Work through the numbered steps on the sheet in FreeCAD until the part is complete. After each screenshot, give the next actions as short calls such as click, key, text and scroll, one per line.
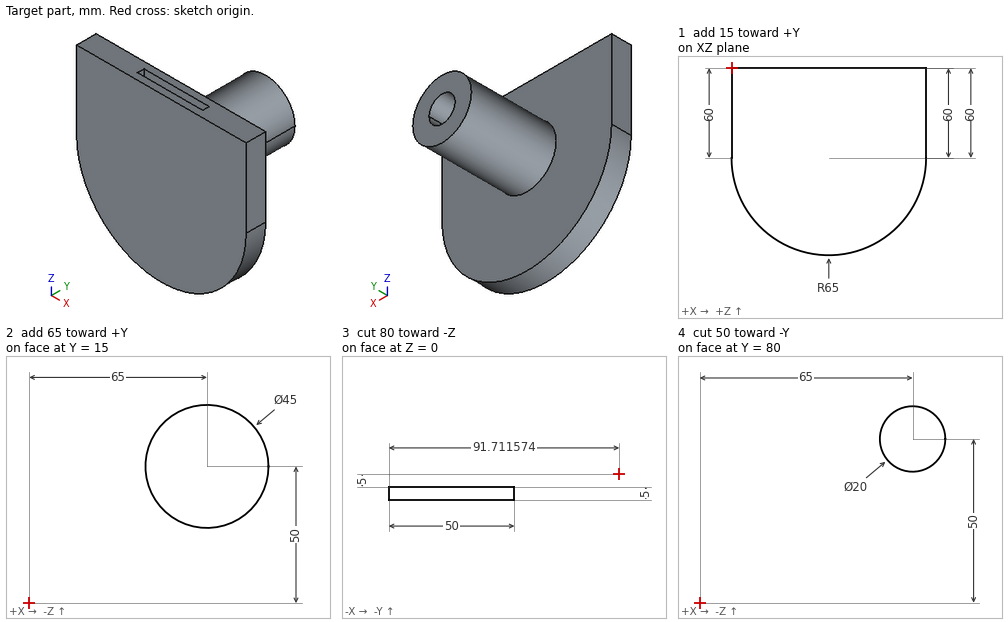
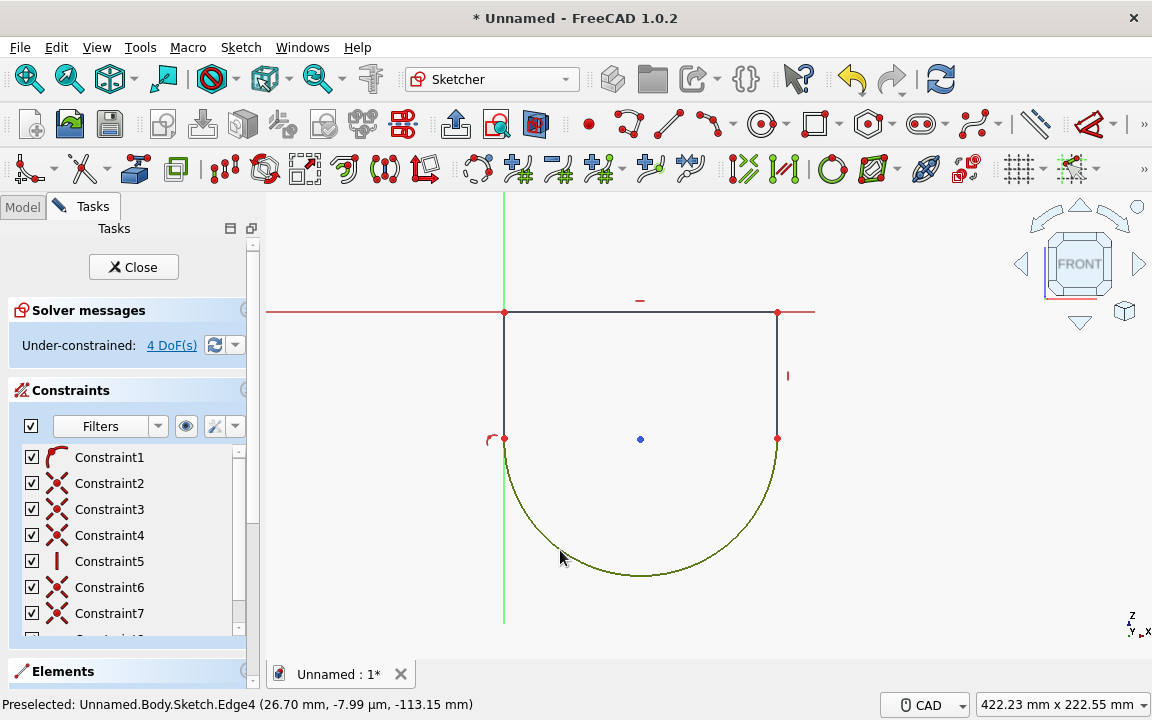
key(k)
key(r)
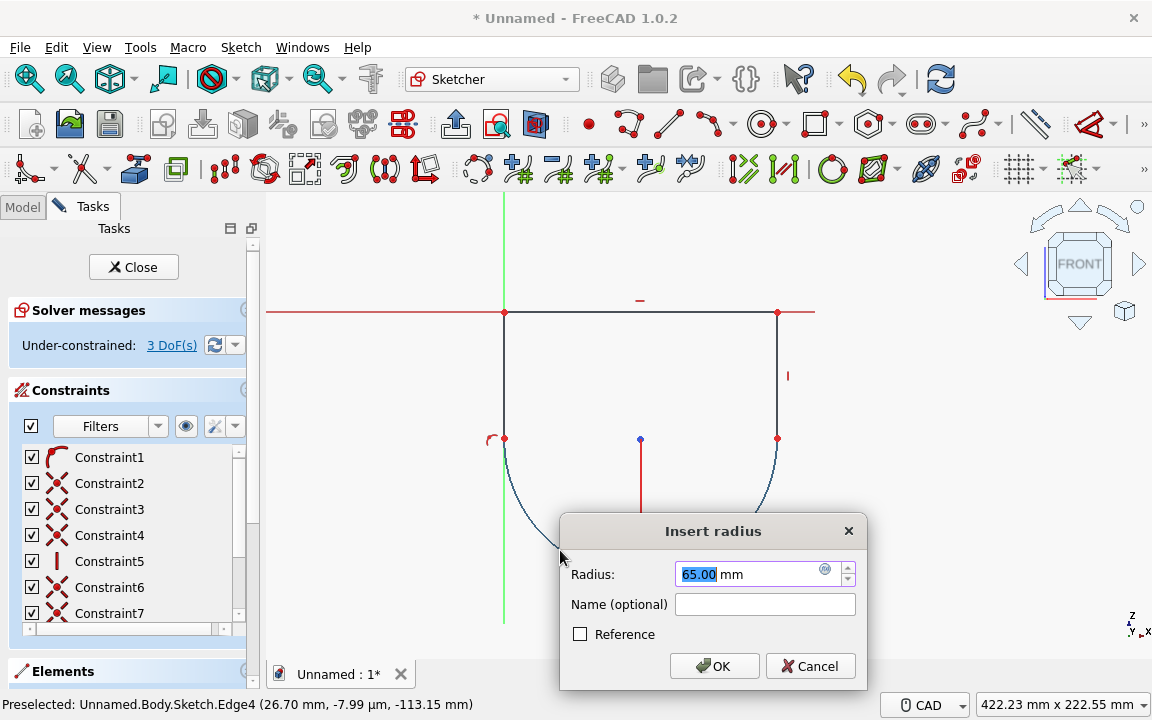
text(65)
key(Return)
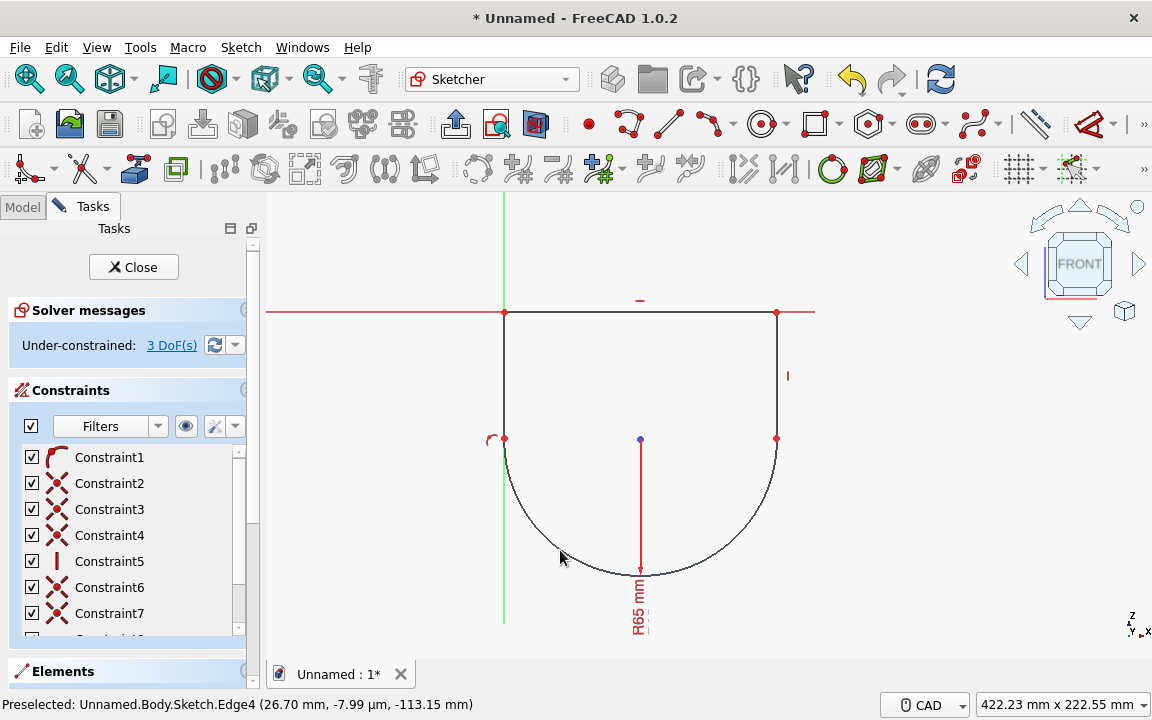
click(504, 401)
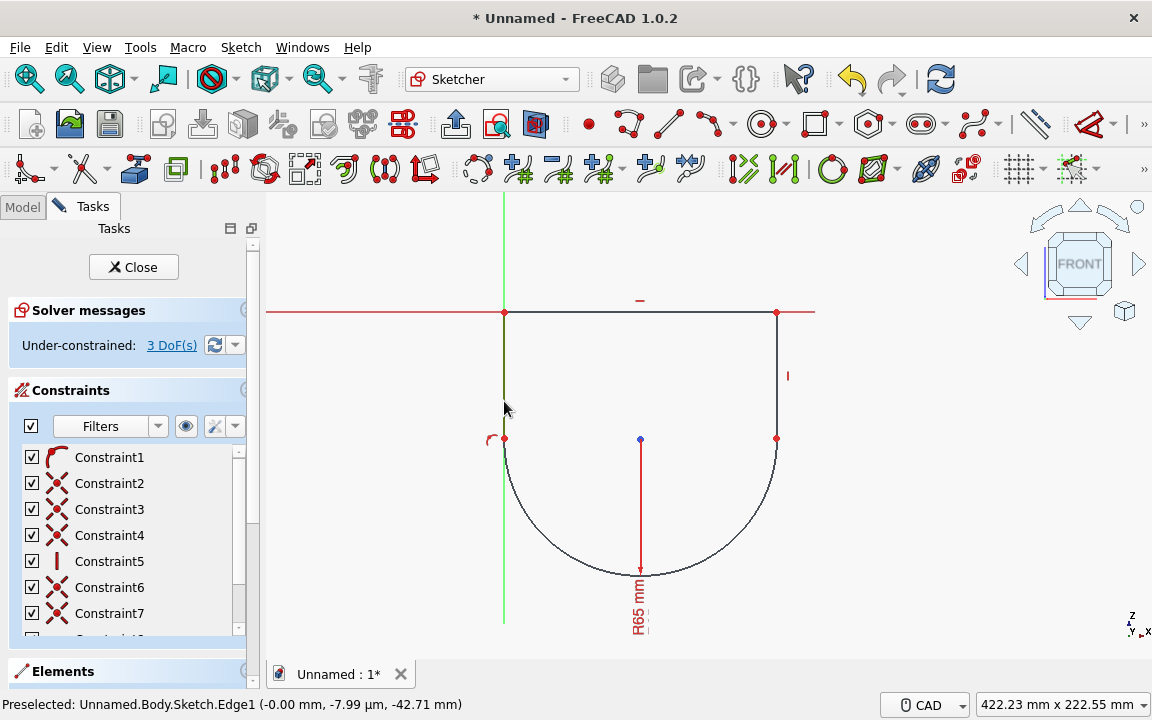
click(1116, 124)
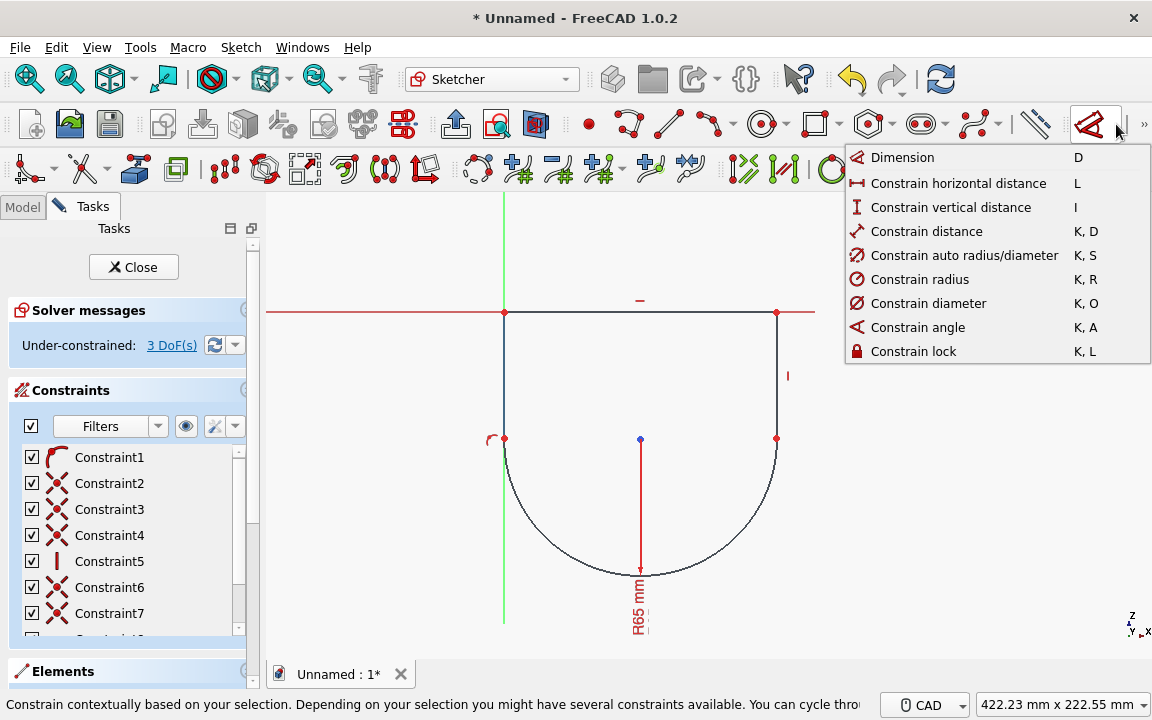
click(998, 207)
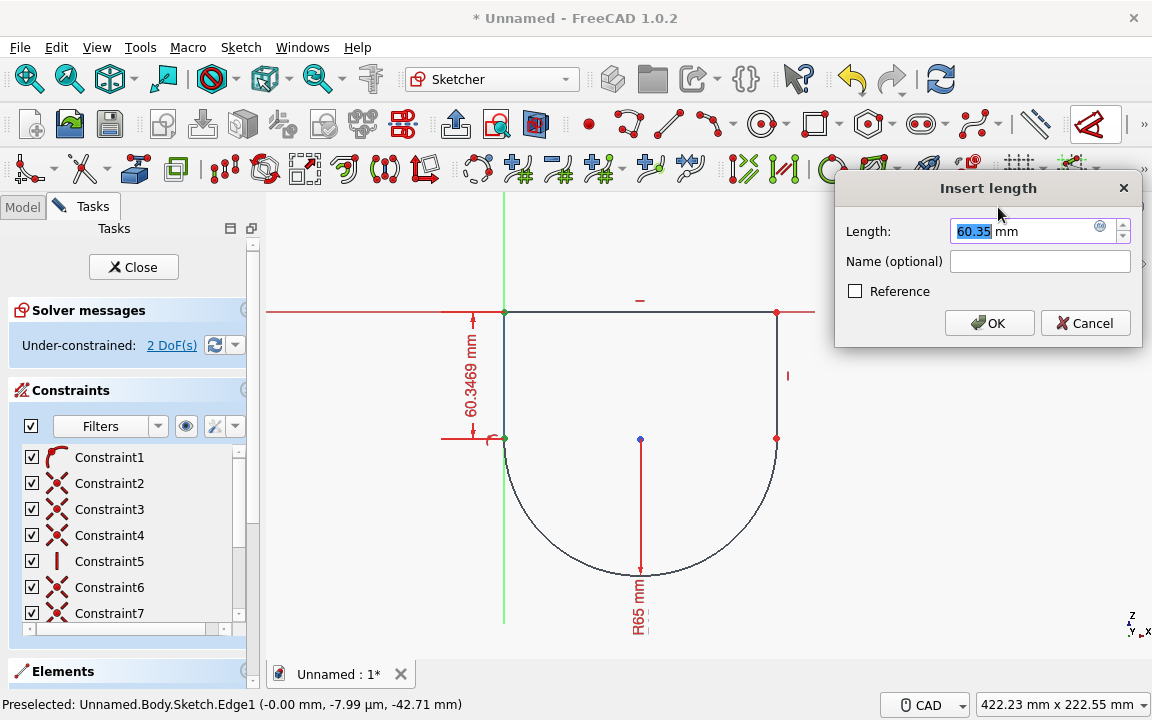
text(60)
key(Return)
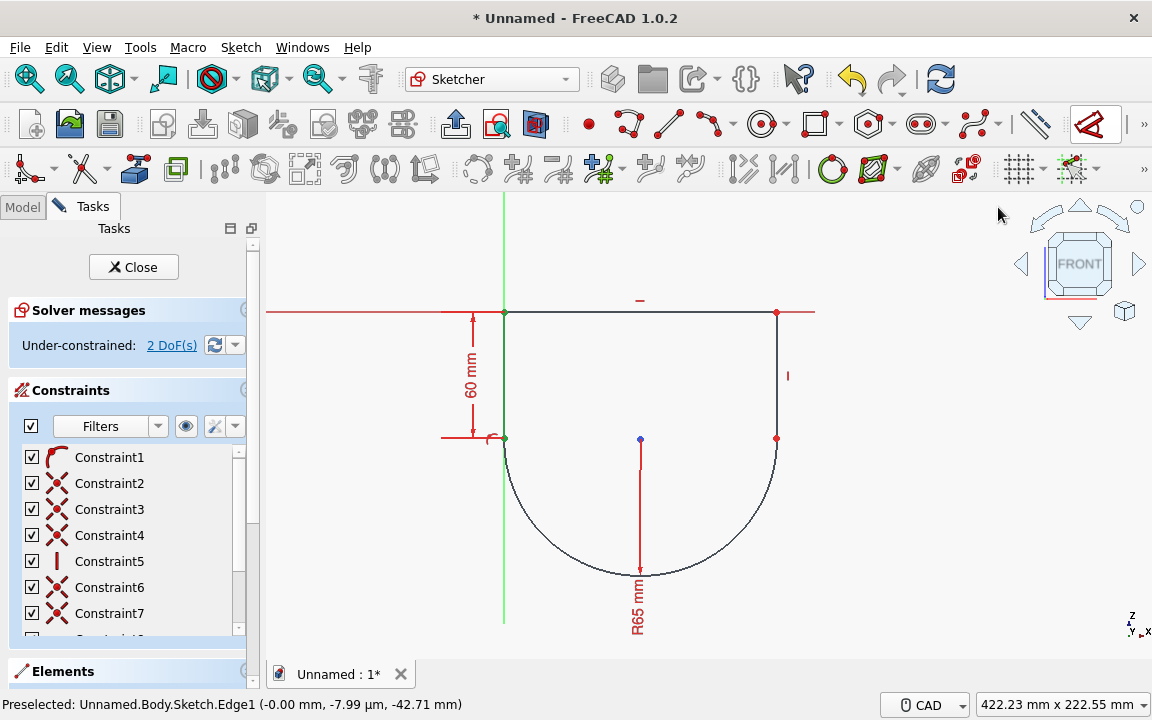
click(777, 350)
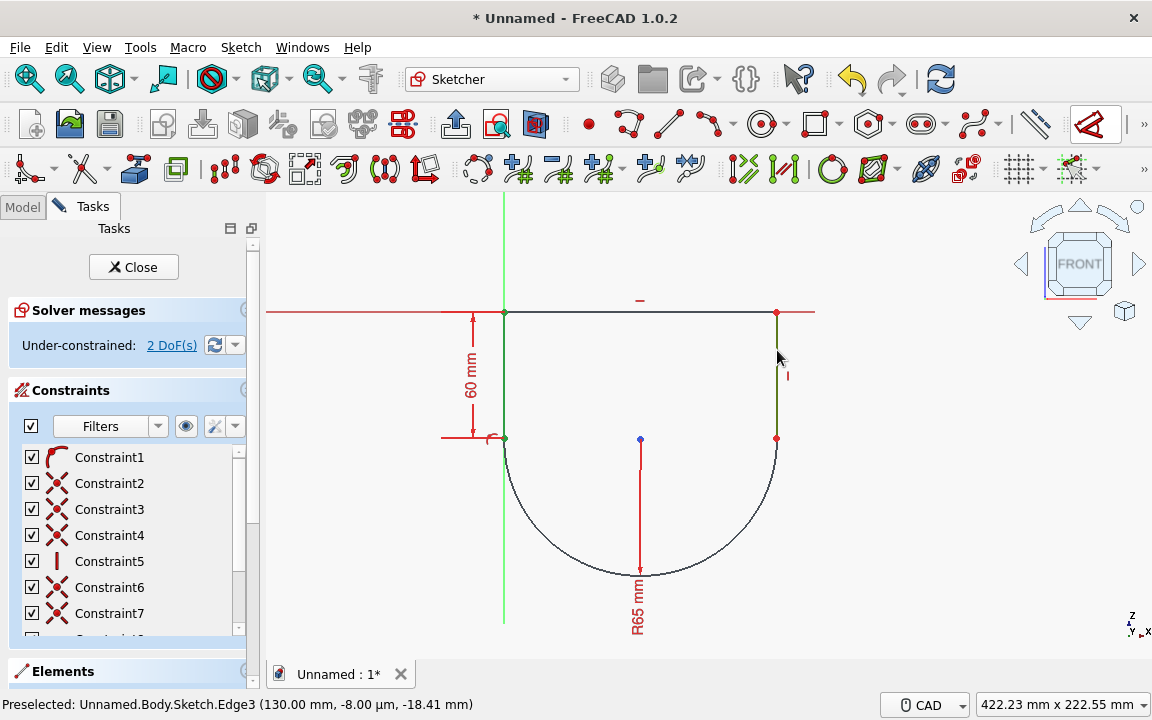
key(i)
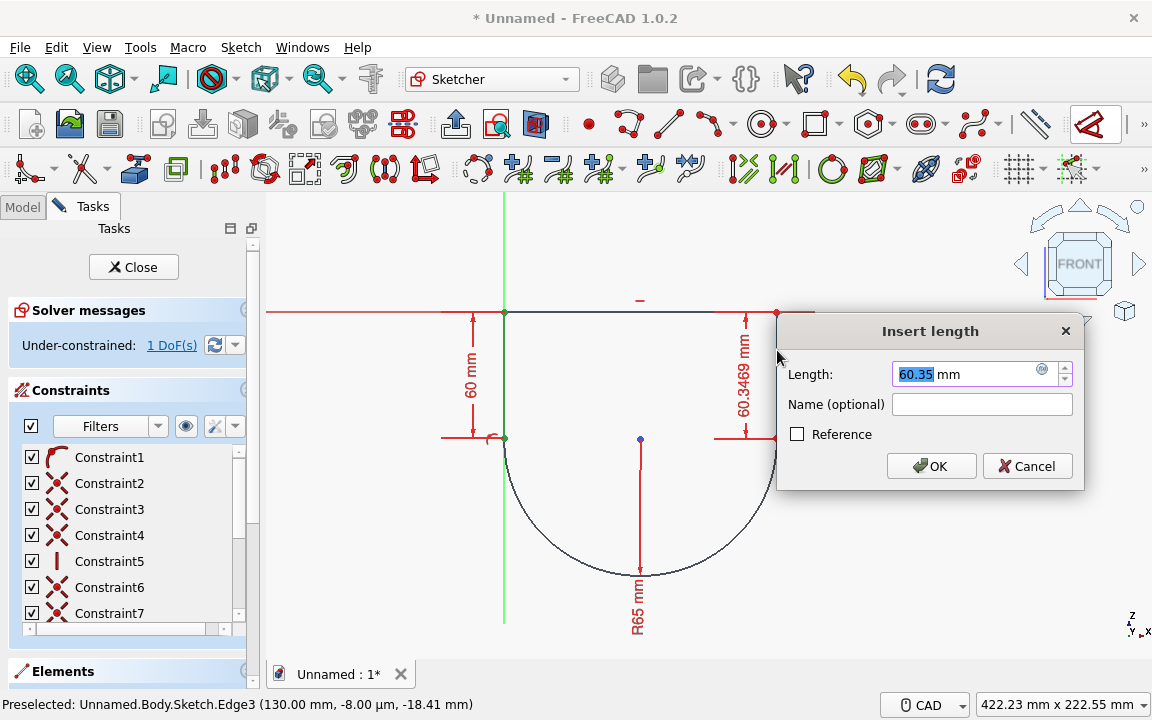
text(60)
key(Return)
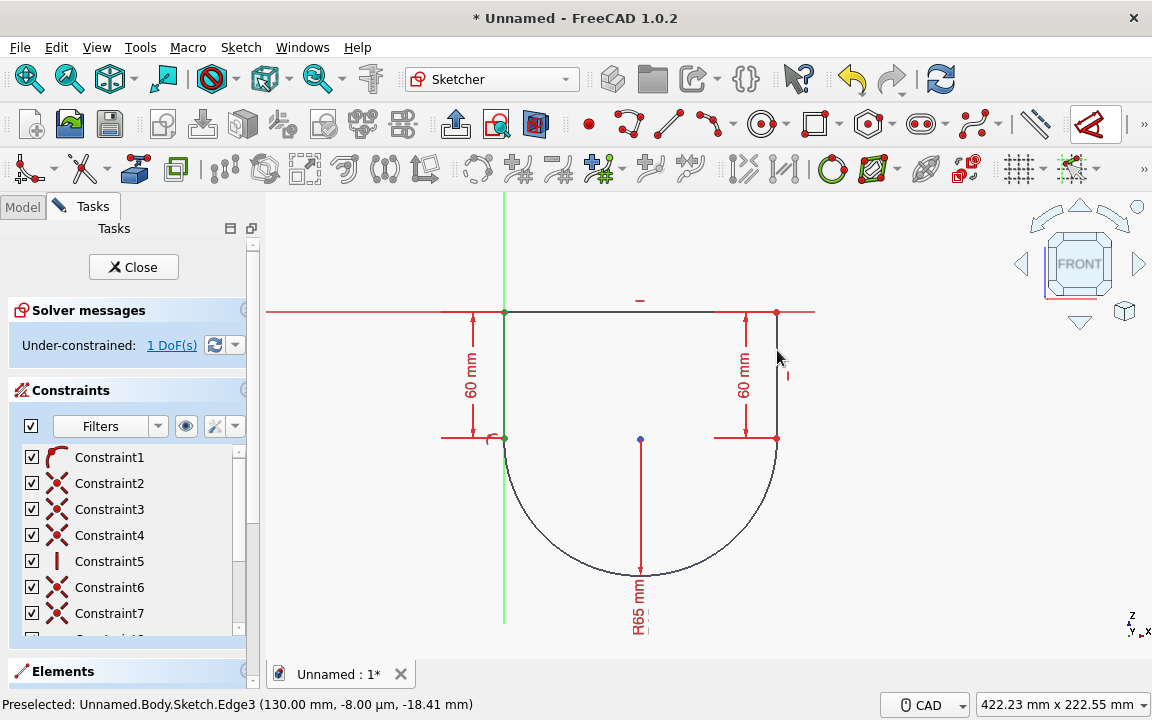
click(641, 440)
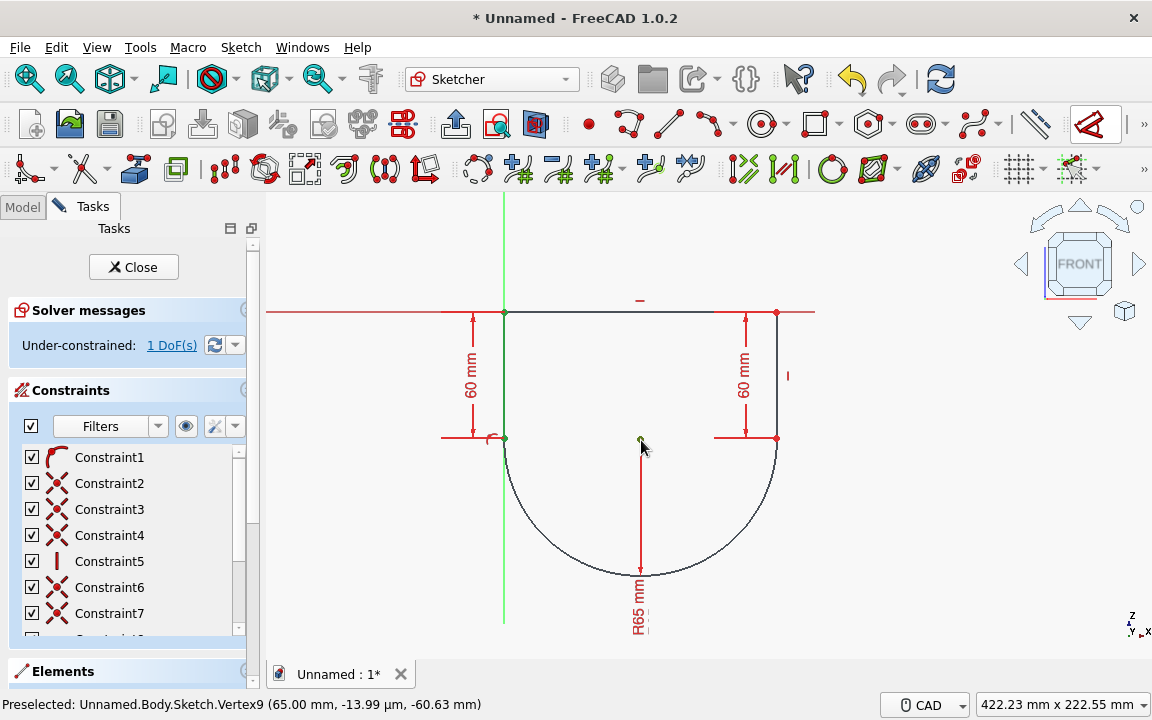
key(i)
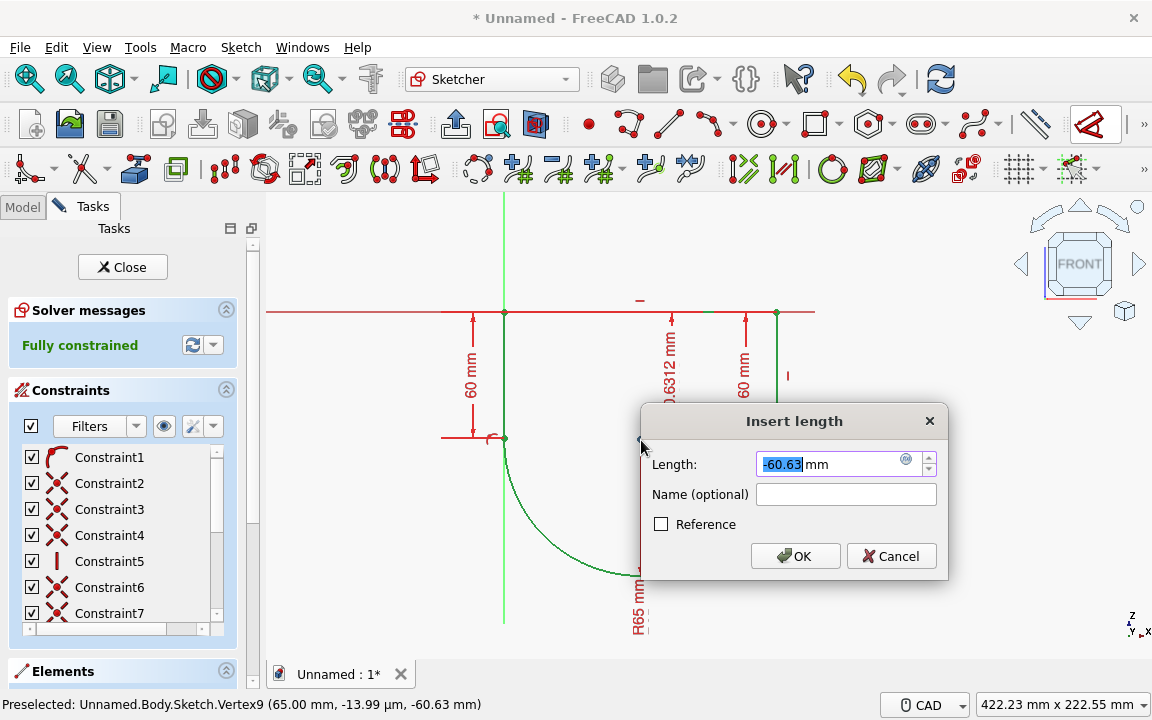
text(-60)
key(Return)